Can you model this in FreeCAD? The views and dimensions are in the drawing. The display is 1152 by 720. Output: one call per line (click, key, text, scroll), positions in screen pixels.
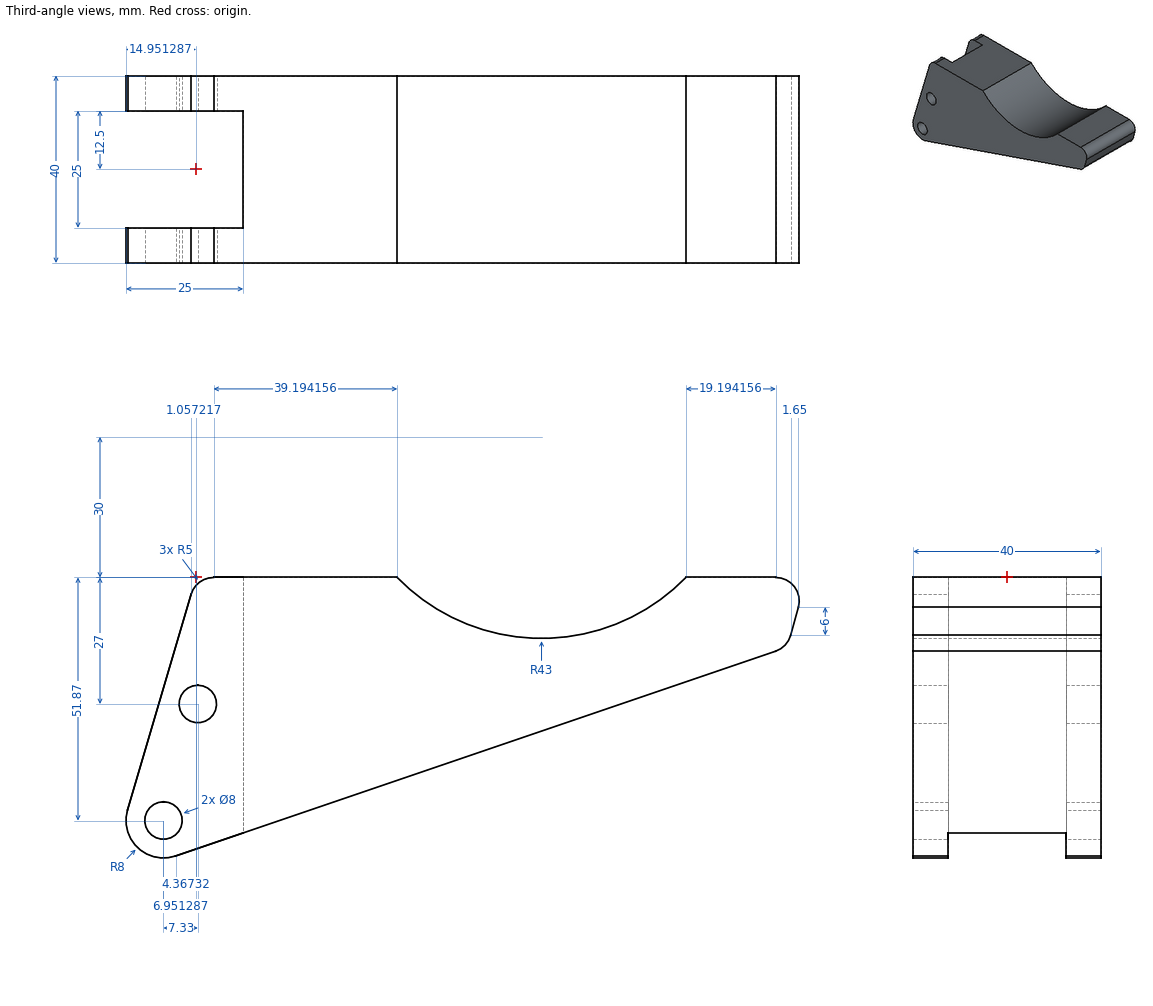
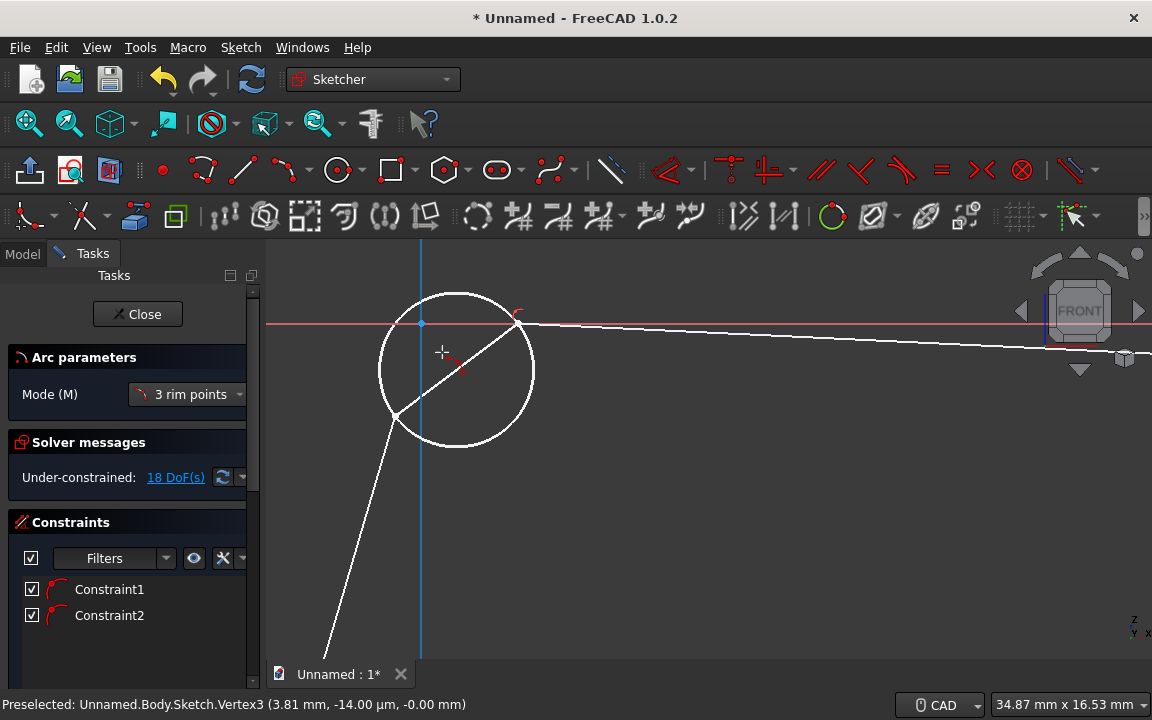
click(440, 349)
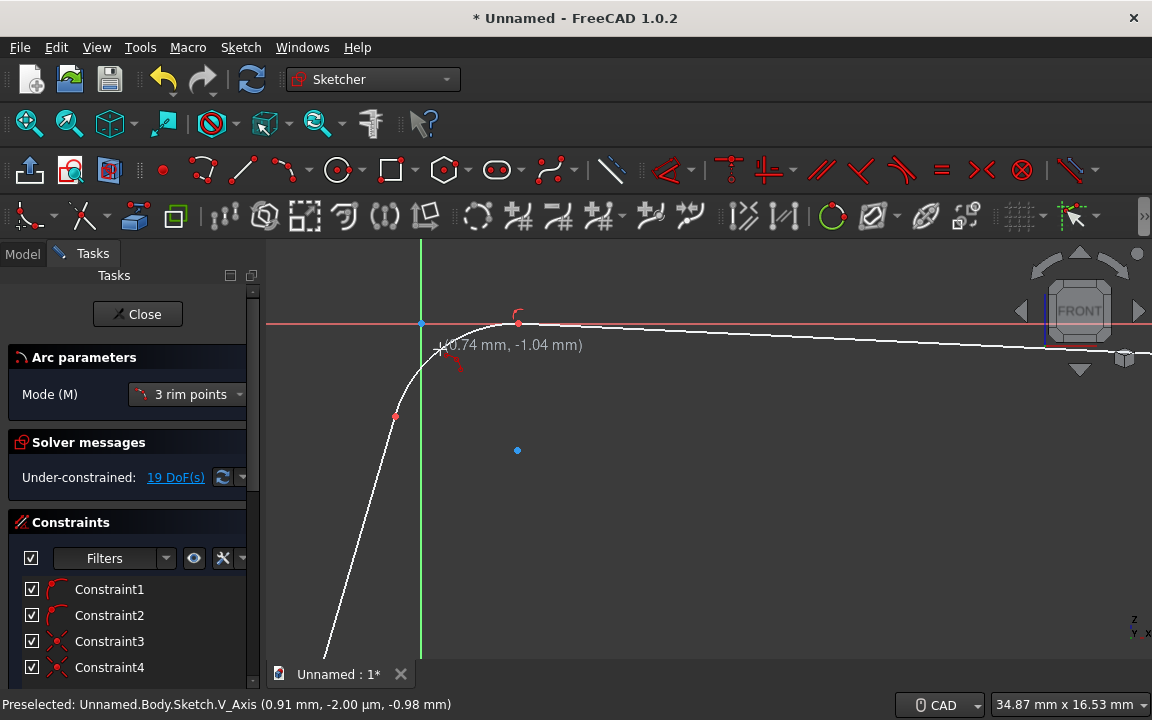
scroll(448, 350, down, 10)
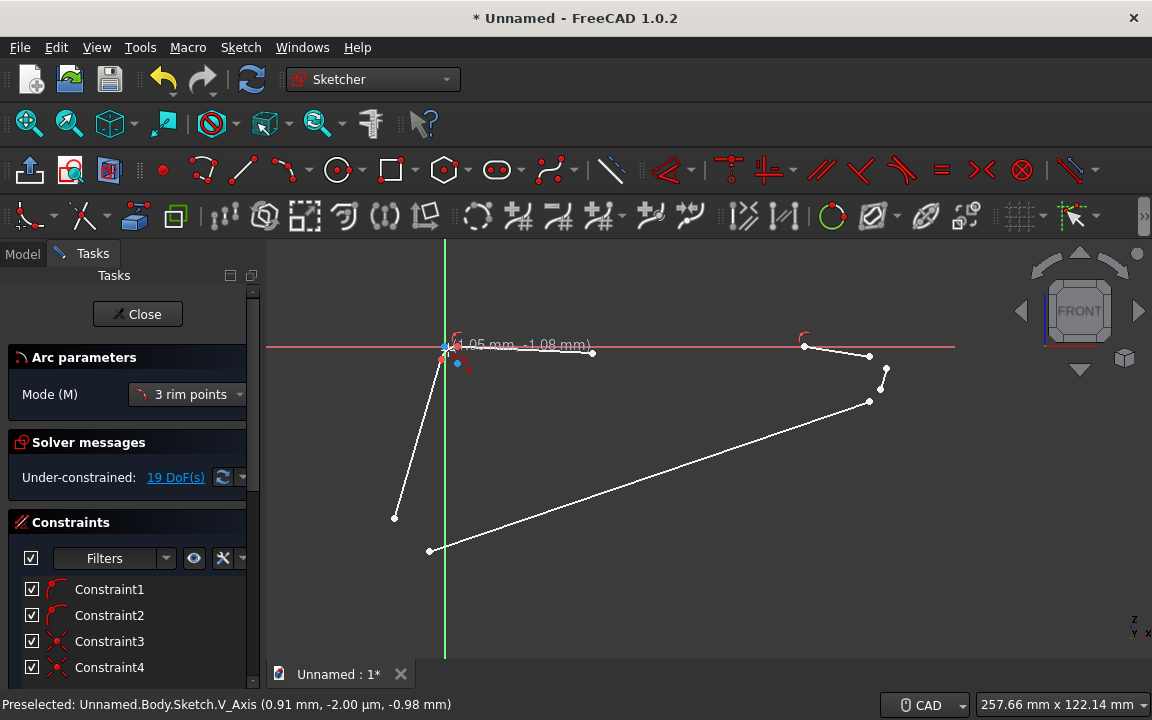
click(592, 353)
click(804, 347)
click(698, 391)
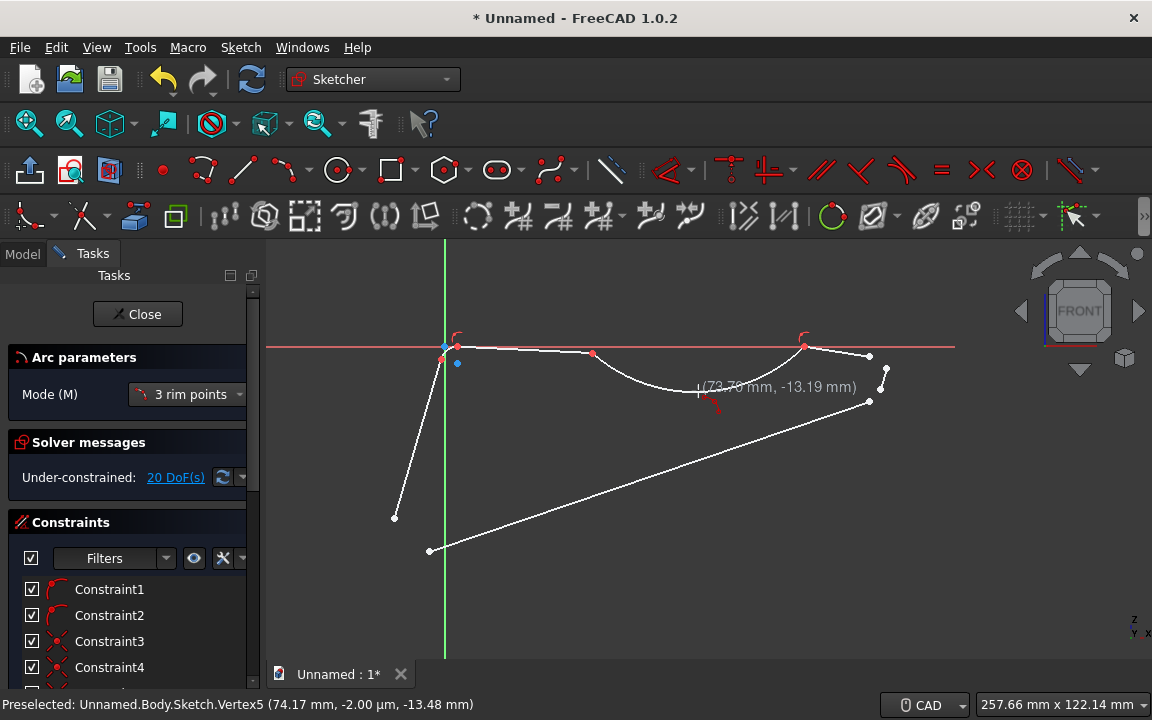
click(870, 357)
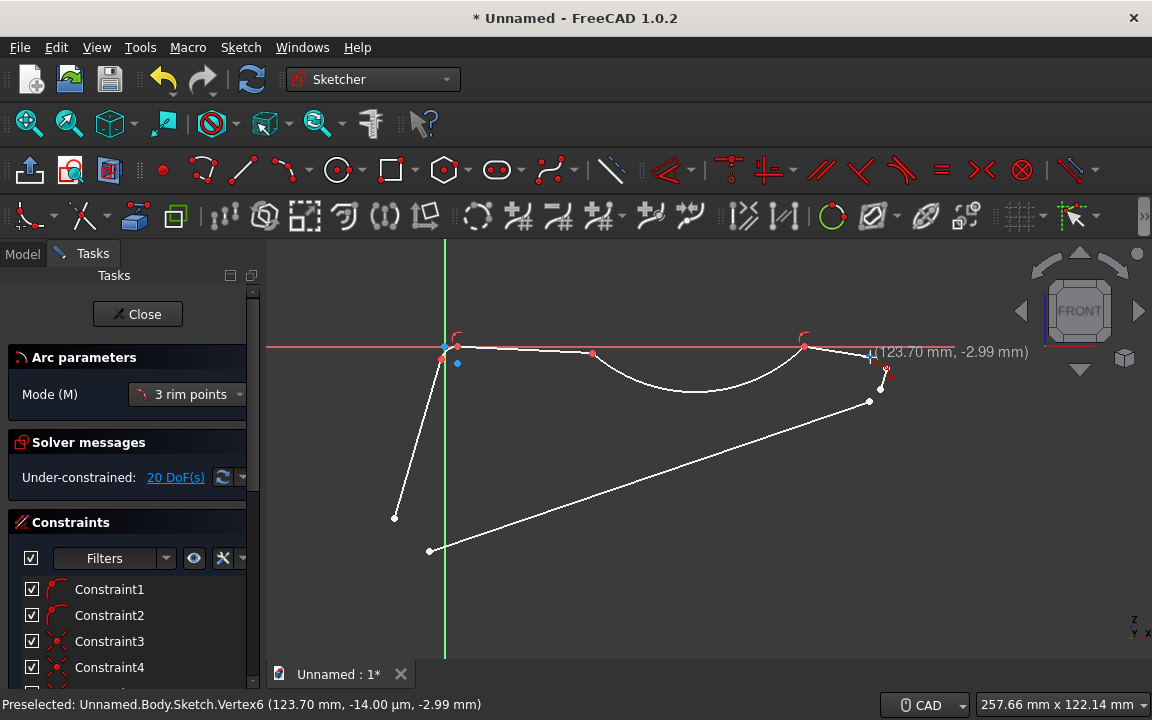
scroll(887, 368, up, 2)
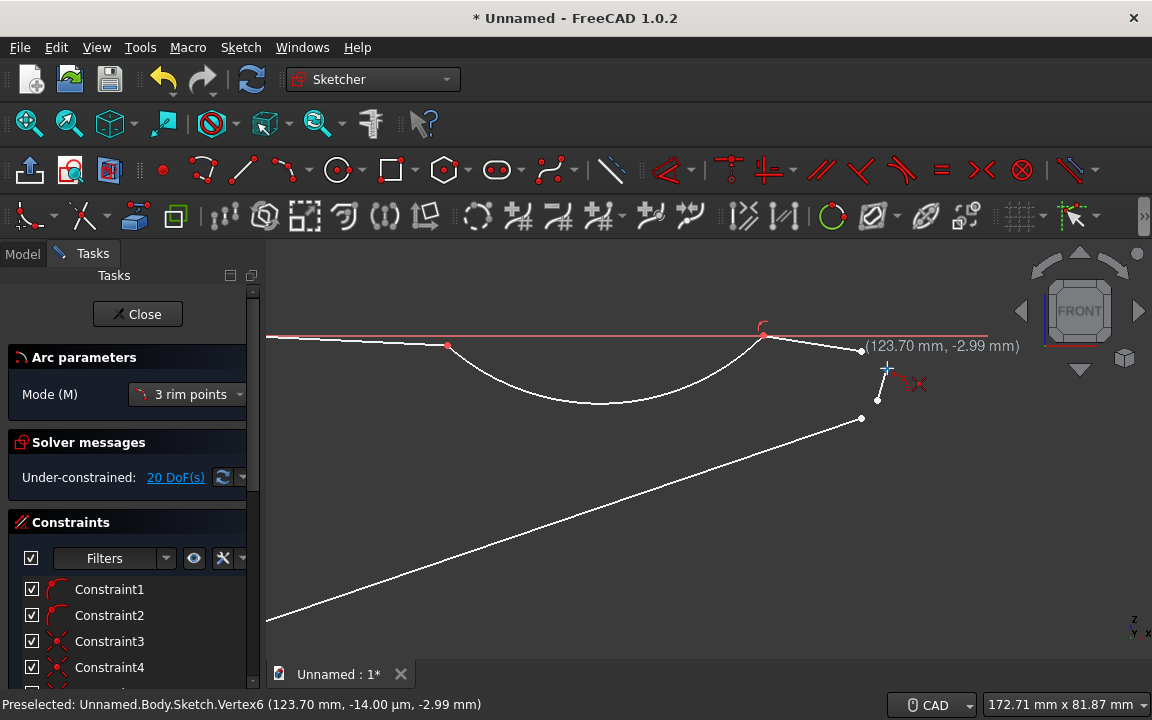
click(887, 369)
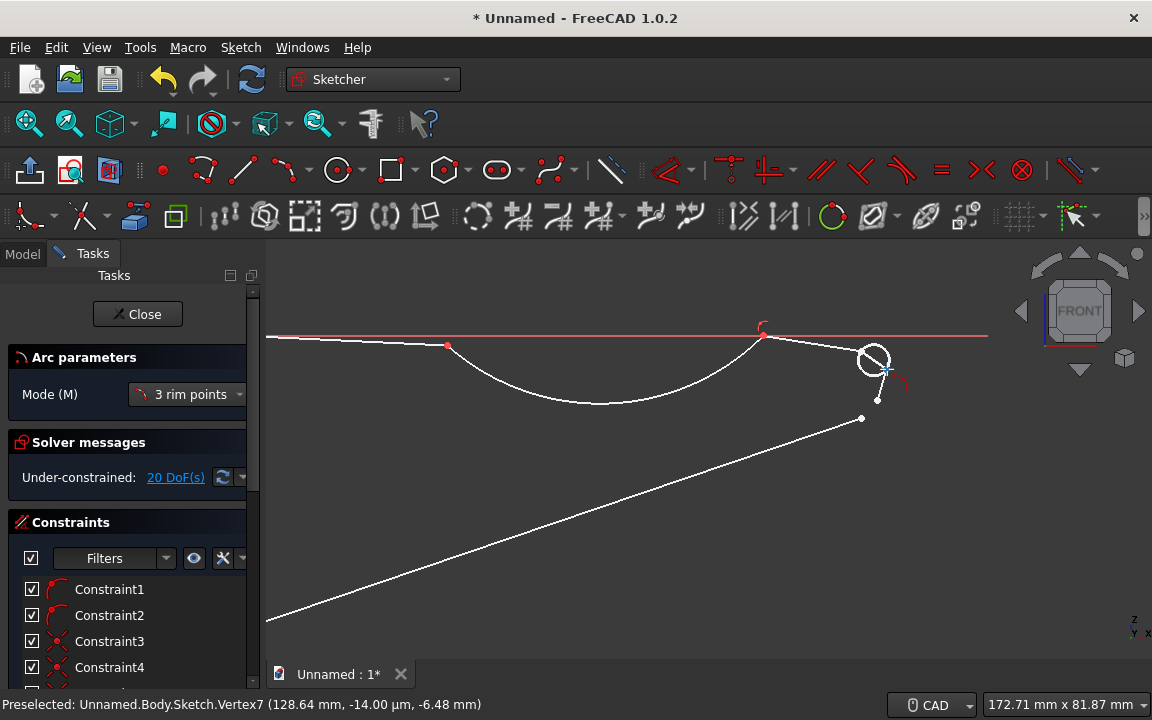
scroll(882, 346, up, 3)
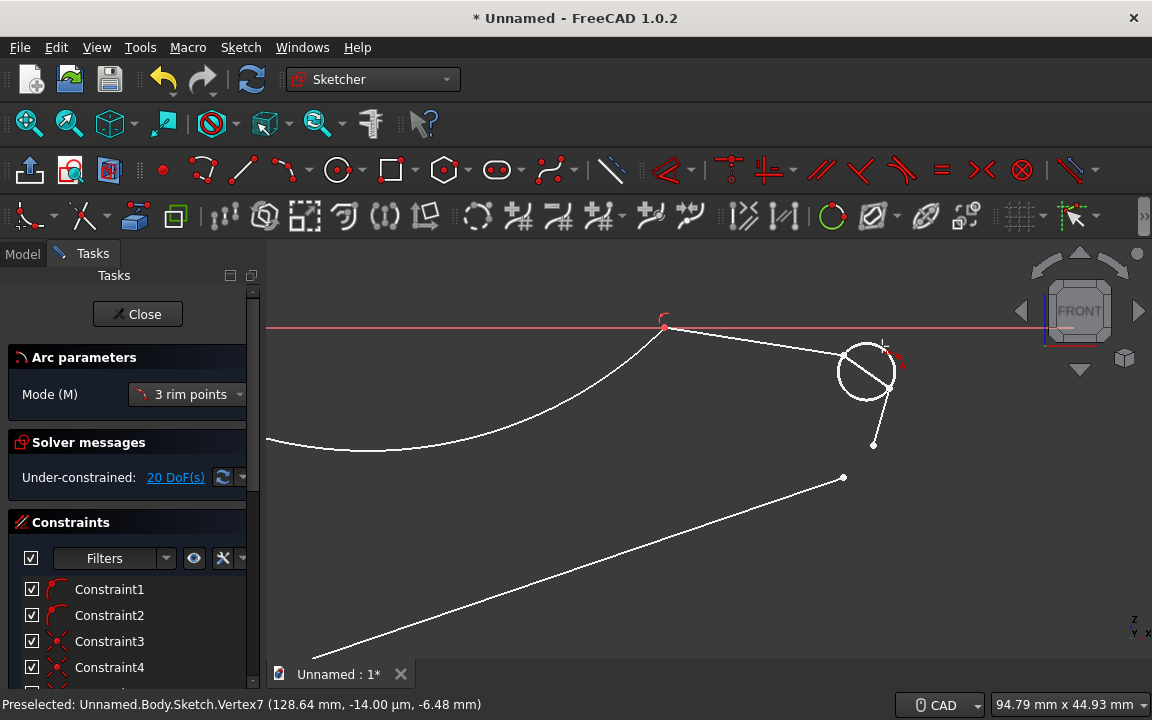
click(881, 346)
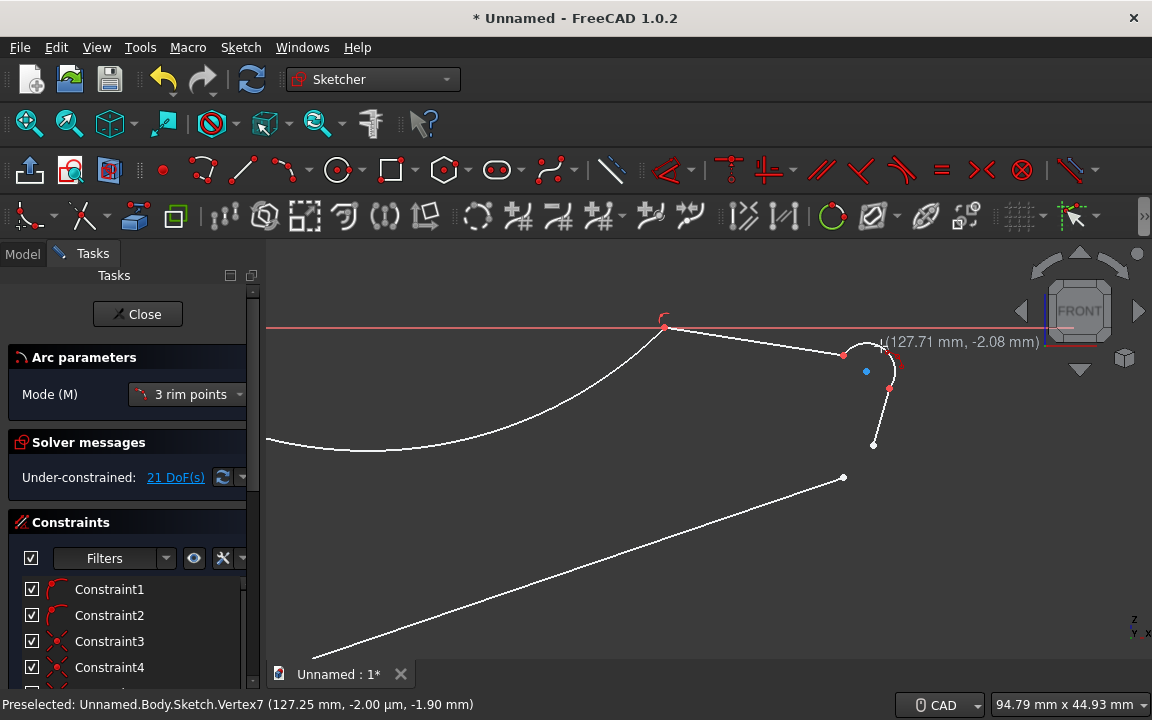
click(873, 445)
click(843, 478)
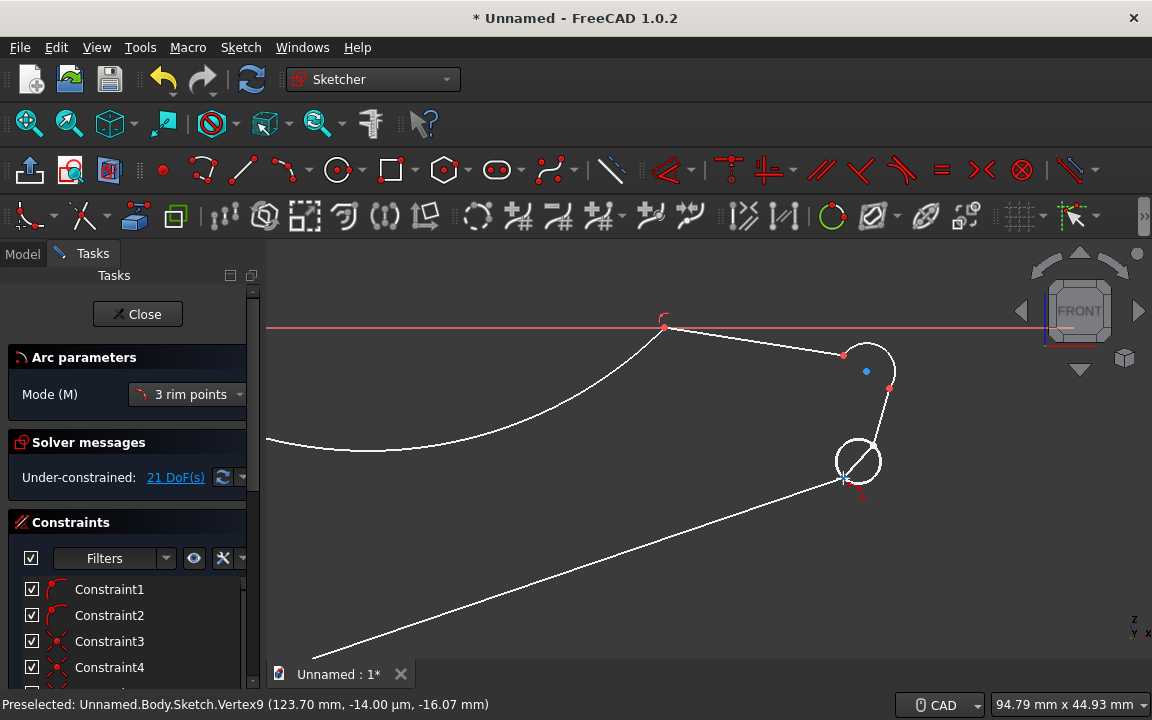
scroll(862, 462, up, 6)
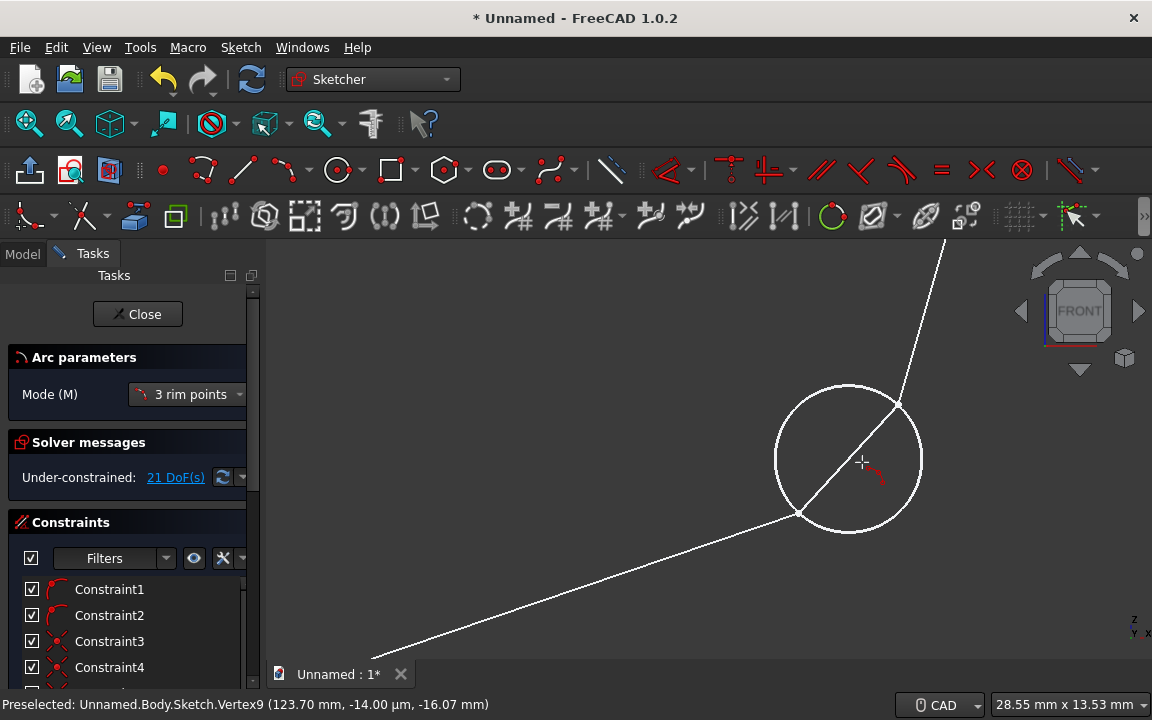
click(862, 462)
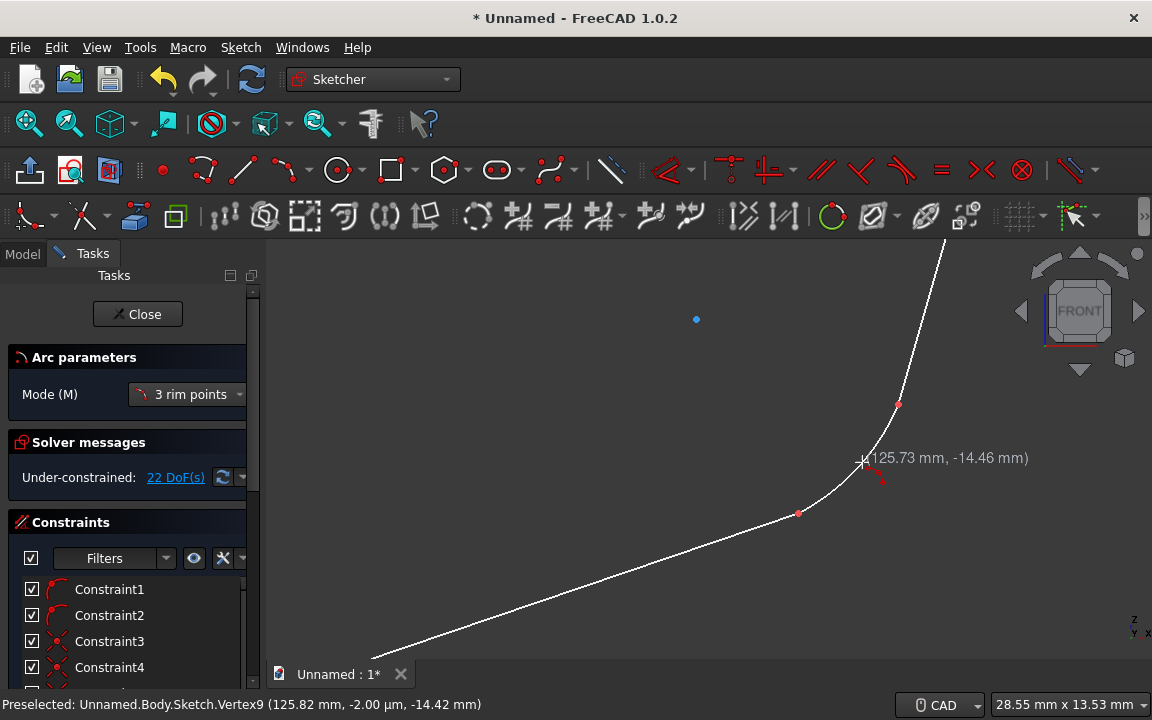
scroll(879, 388, down, 11)